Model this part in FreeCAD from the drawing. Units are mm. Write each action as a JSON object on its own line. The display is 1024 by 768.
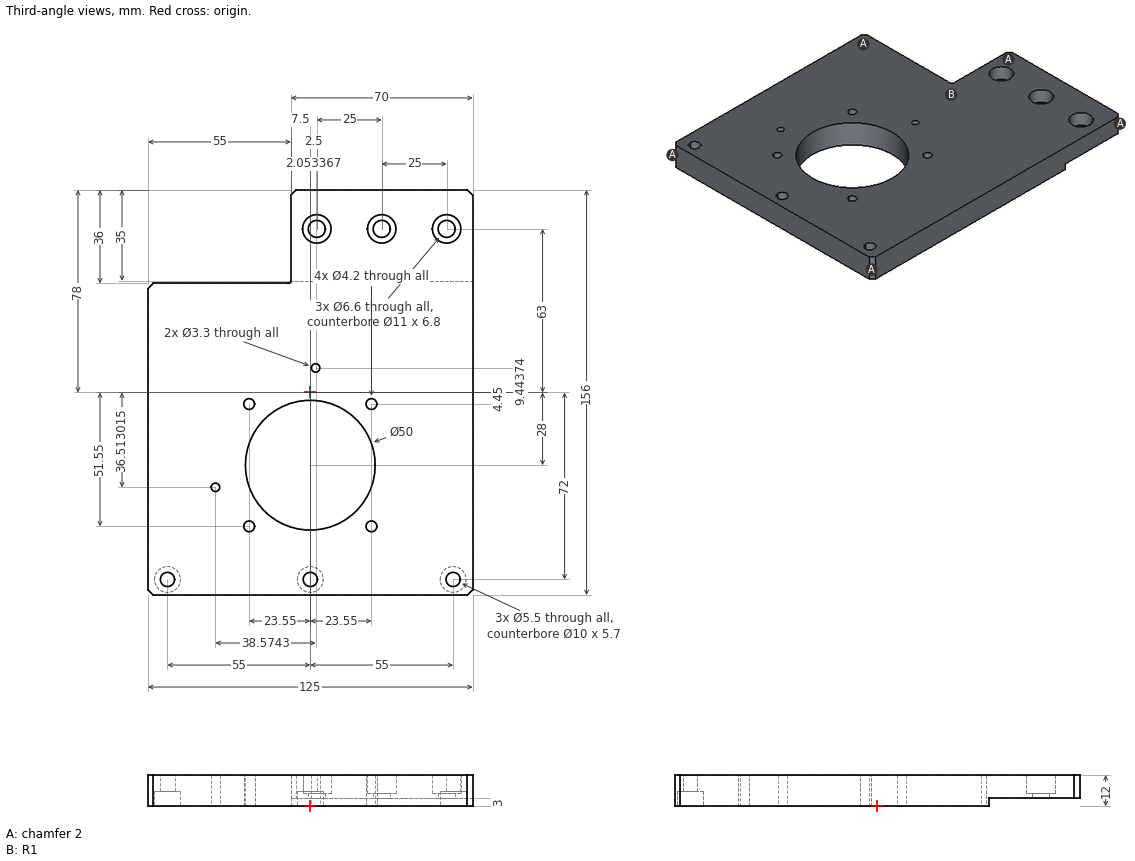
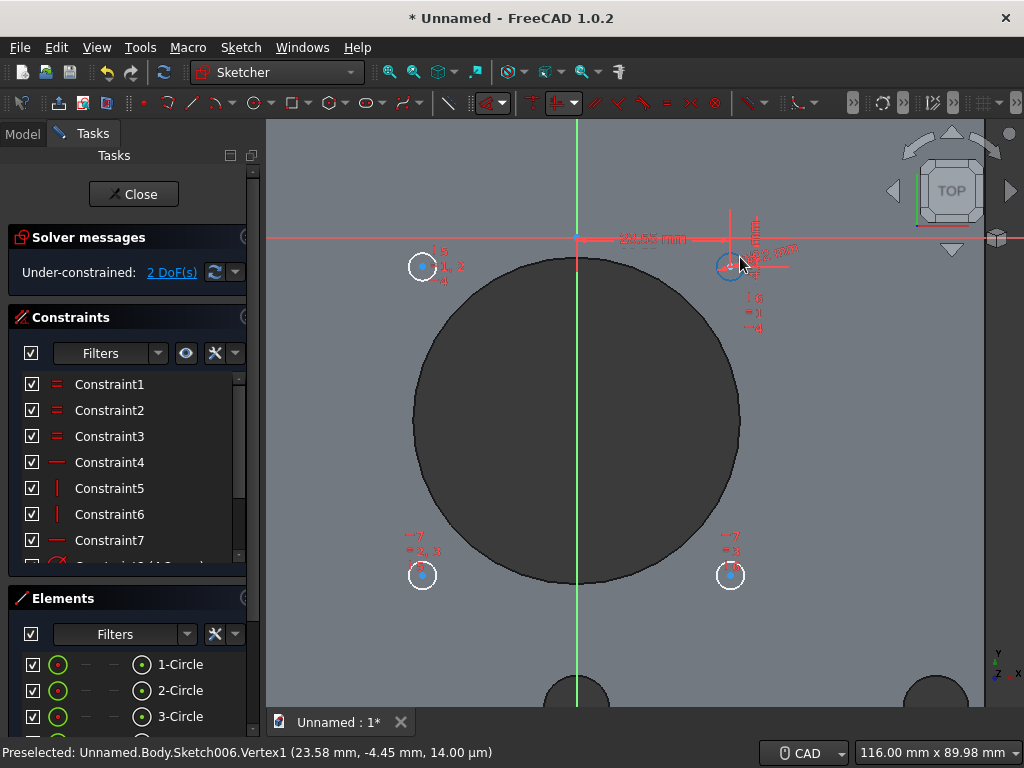
{"action": "left_click", "coordinate": [423, 267]}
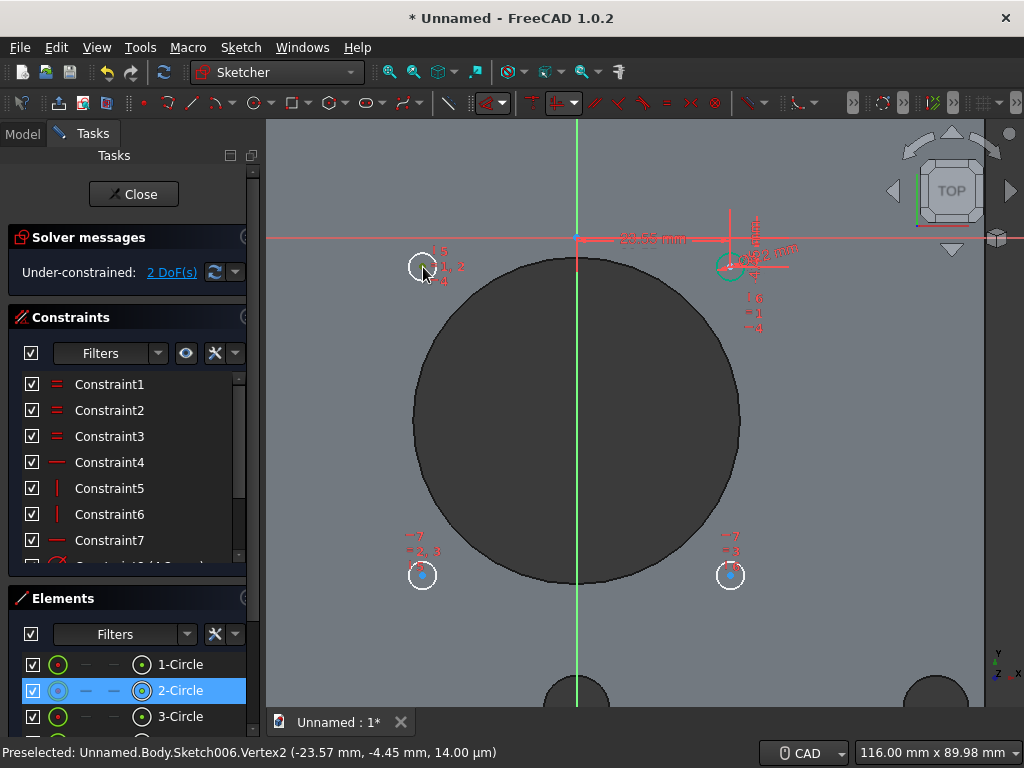
{"action": "left_click", "coordinate": [504, 104]}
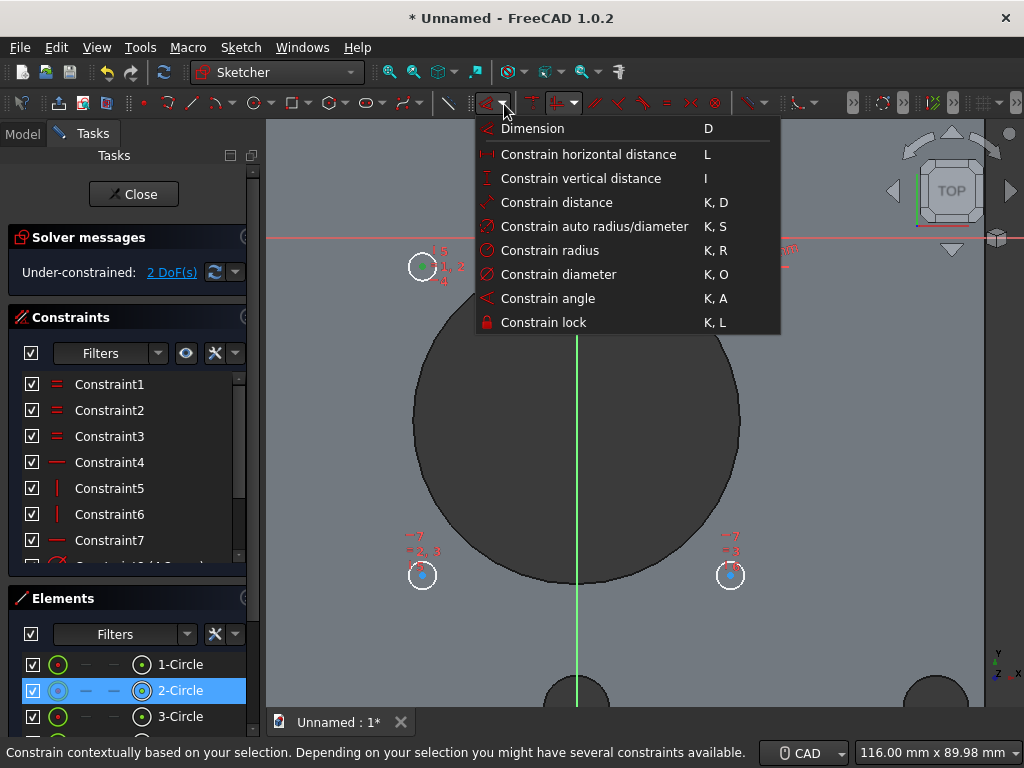
{"action": "left_click", "coordinate": [628, 154]}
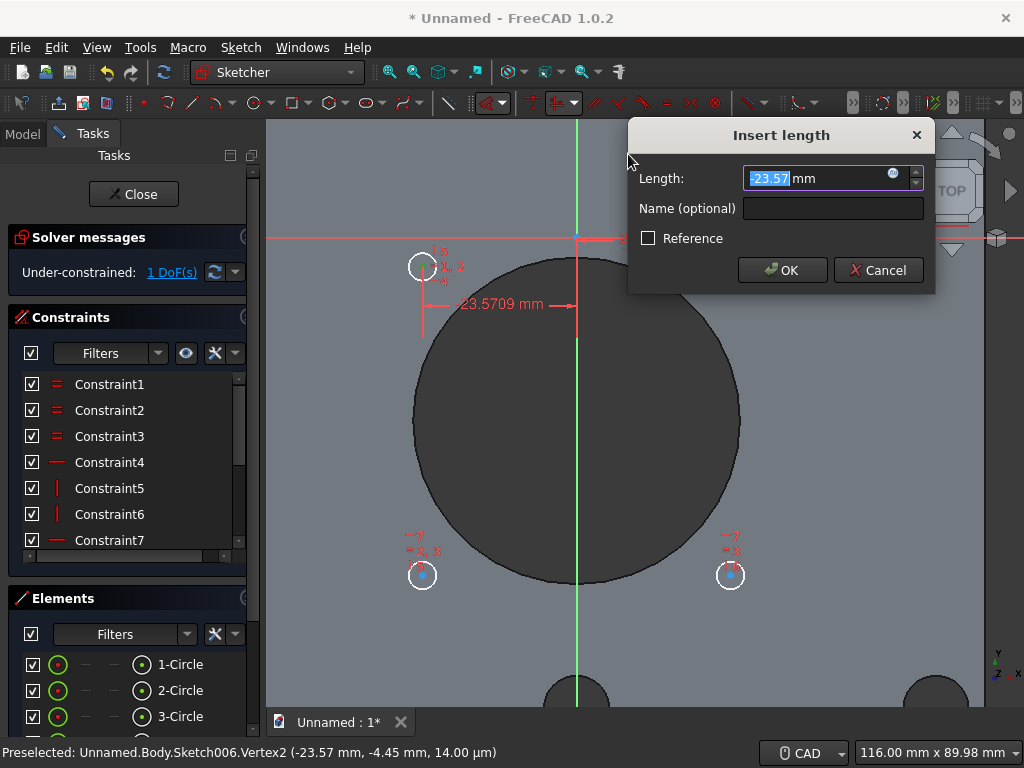
{"action": "type", "text": "-23.55"}
{"action": "key", "text": "Return"}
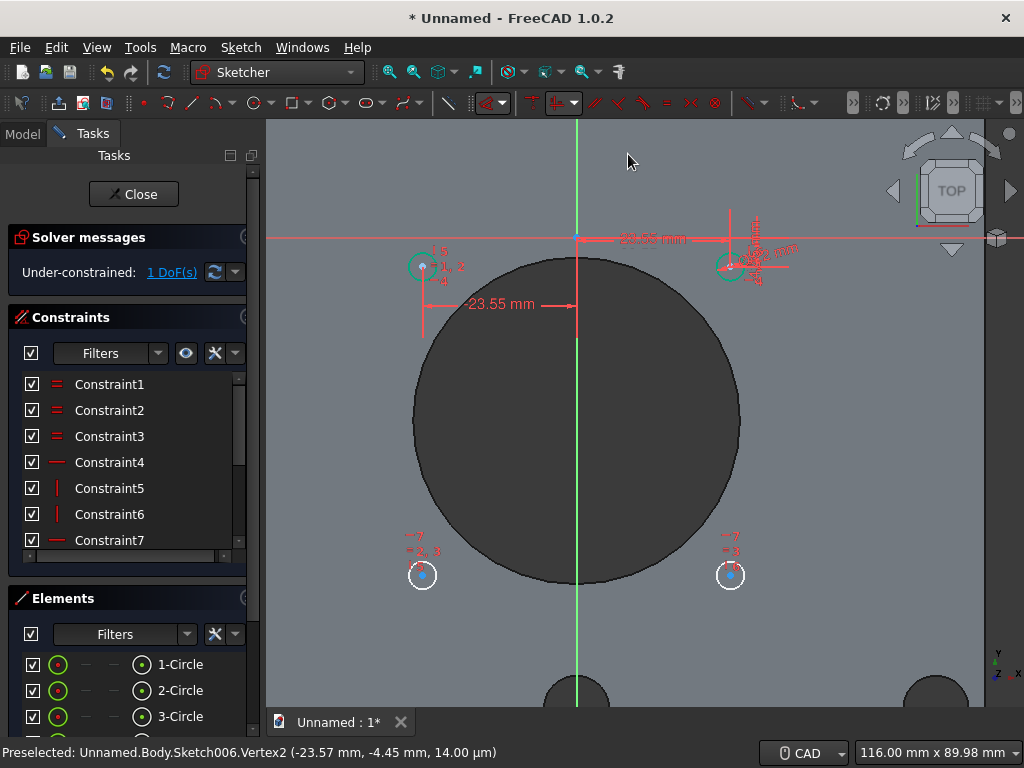
{"action": "left_click", "coordinate": [423, 575]}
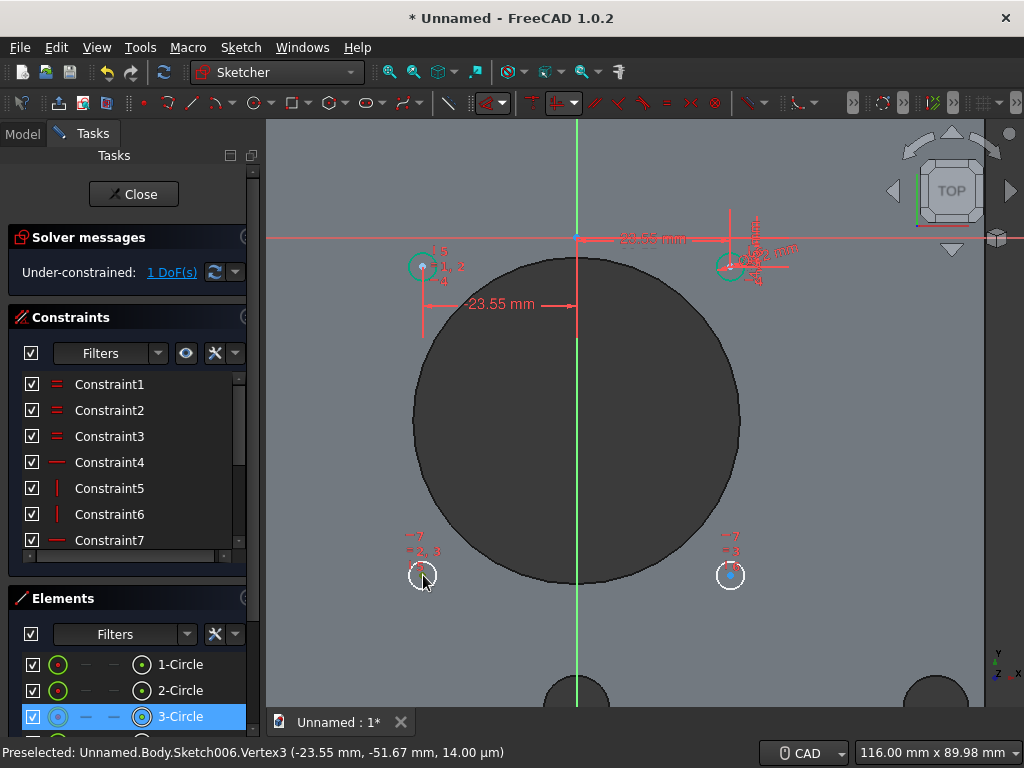
{"action": "left_click", "coordinate": [504, 104]}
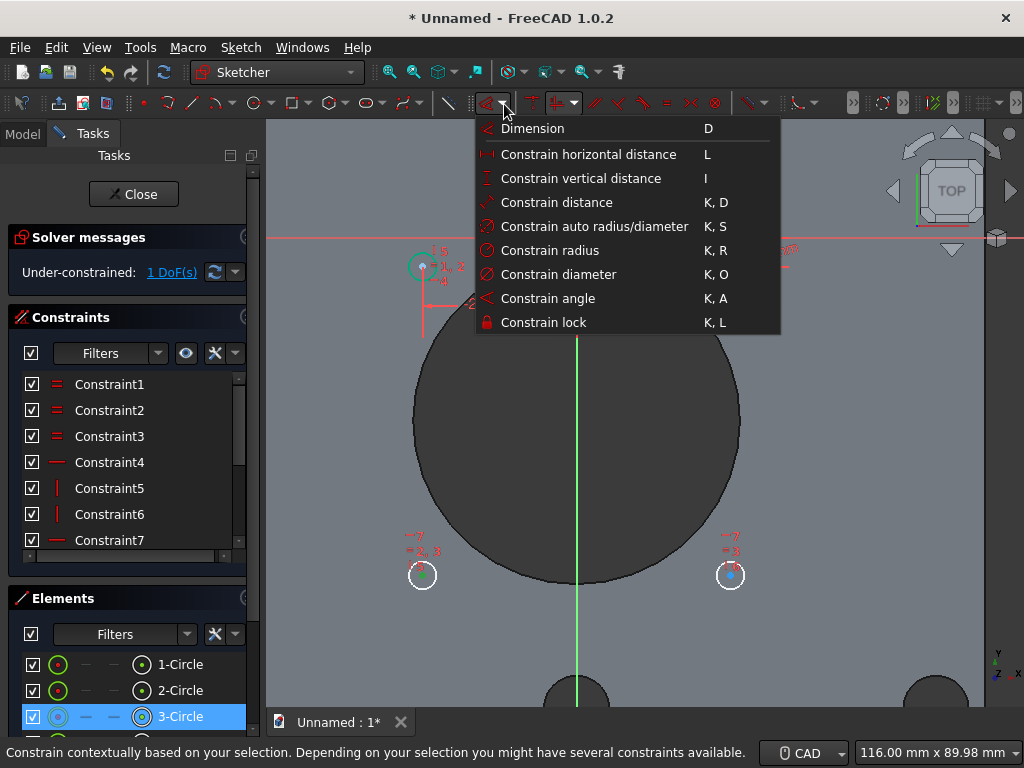
{"action": "left_click", "coordinate": [628, 178]}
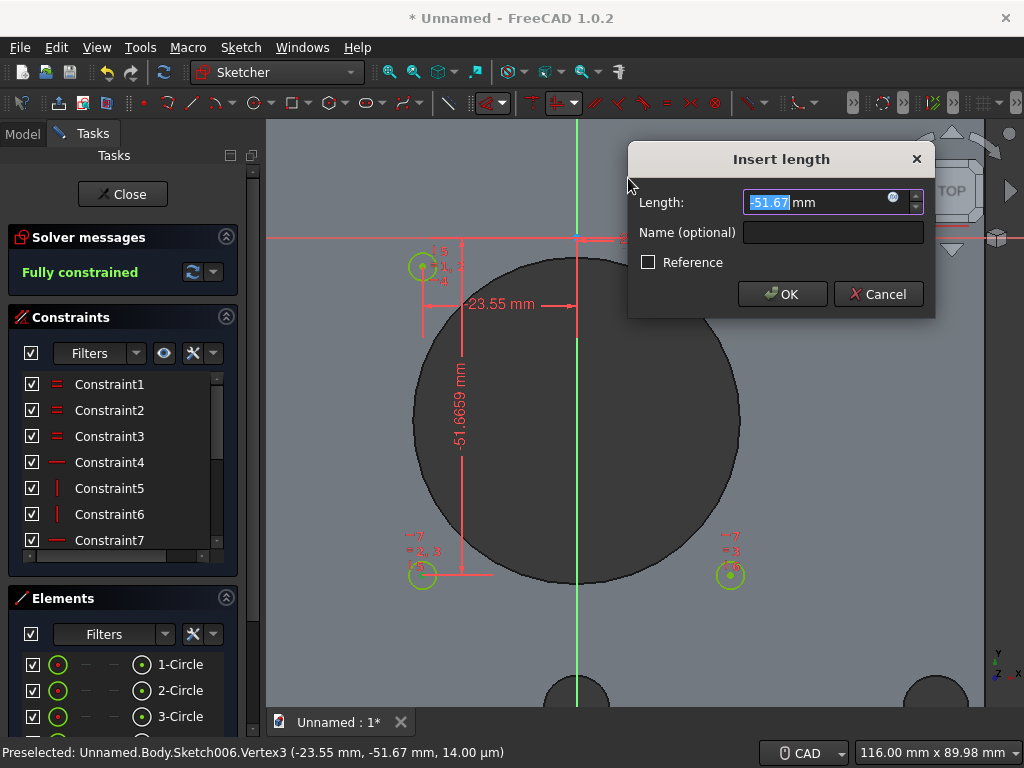
{"action": "type", "text": "-51.55"}
{"action": "key", "text": "Return"}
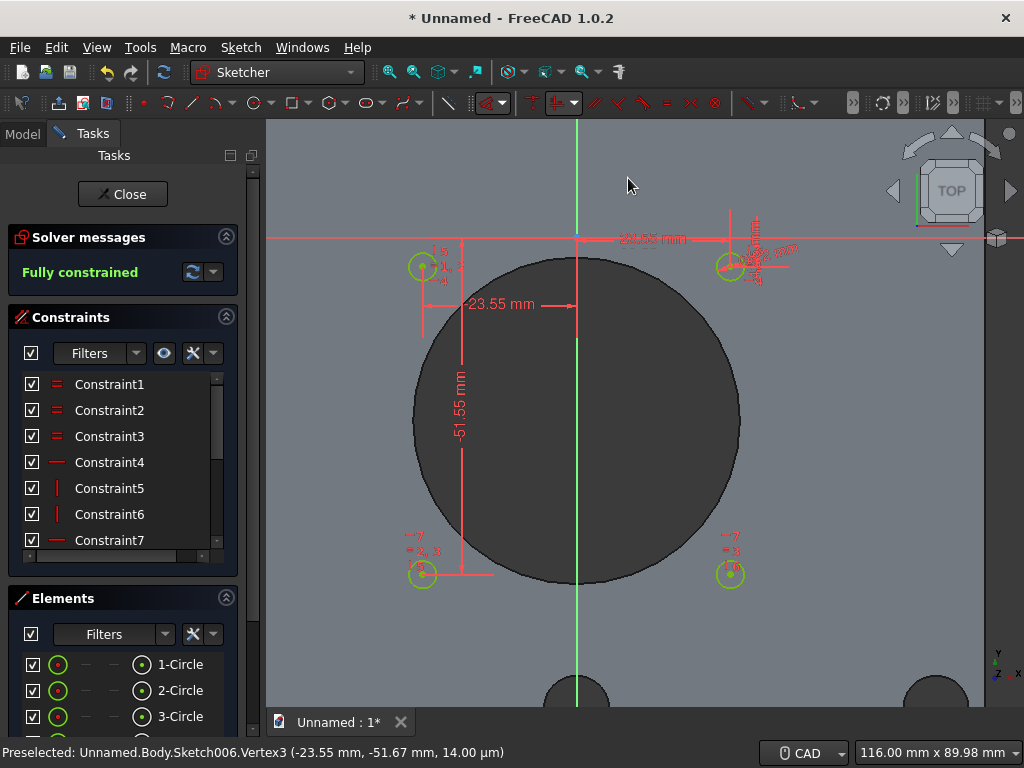
{"action": "left_click", "coordinate": [123, 194]}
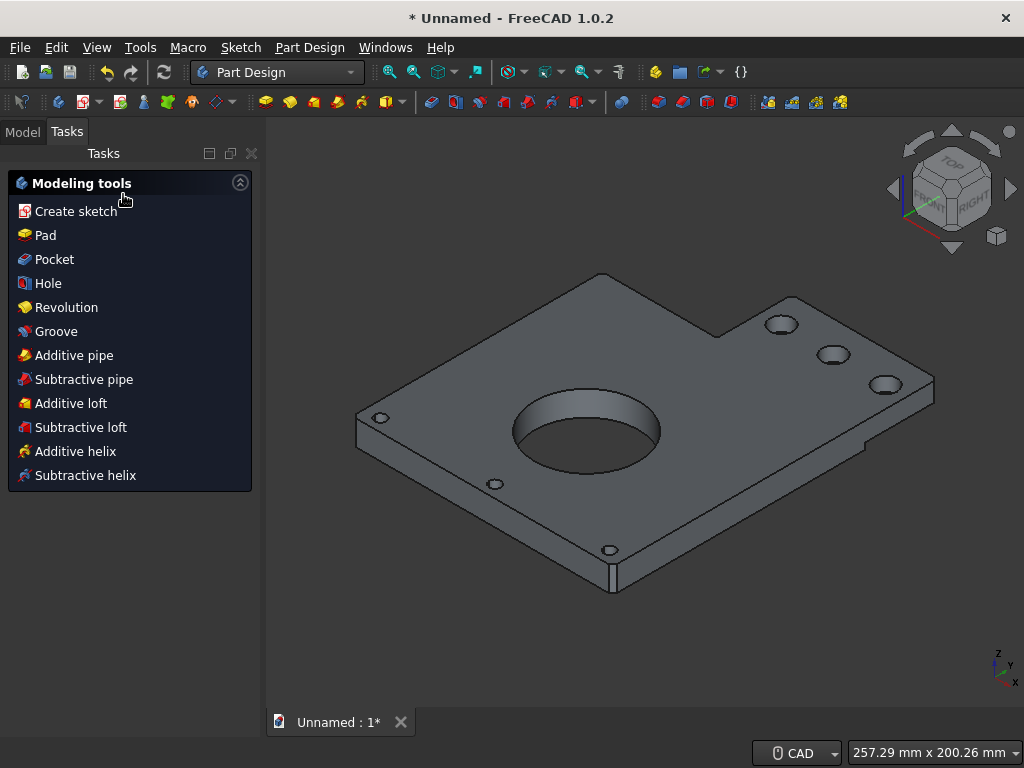
{"action": "left_click", "coordinate": [456, 102]}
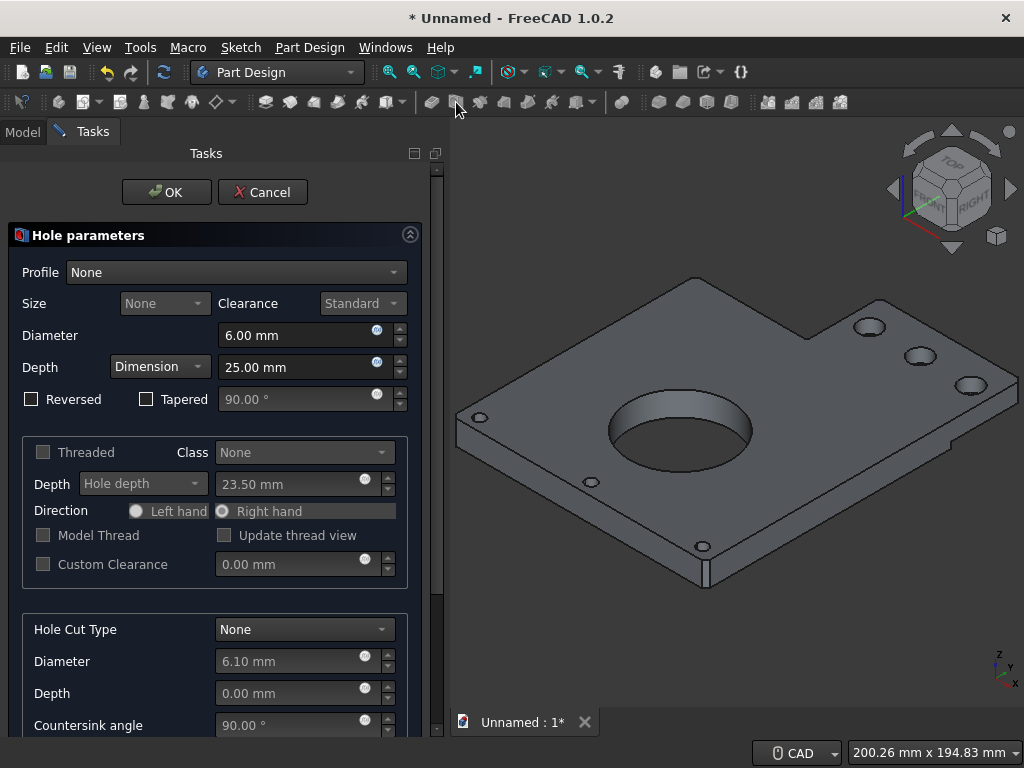
{"action": "triple_click", "coordinate": [305, 335]}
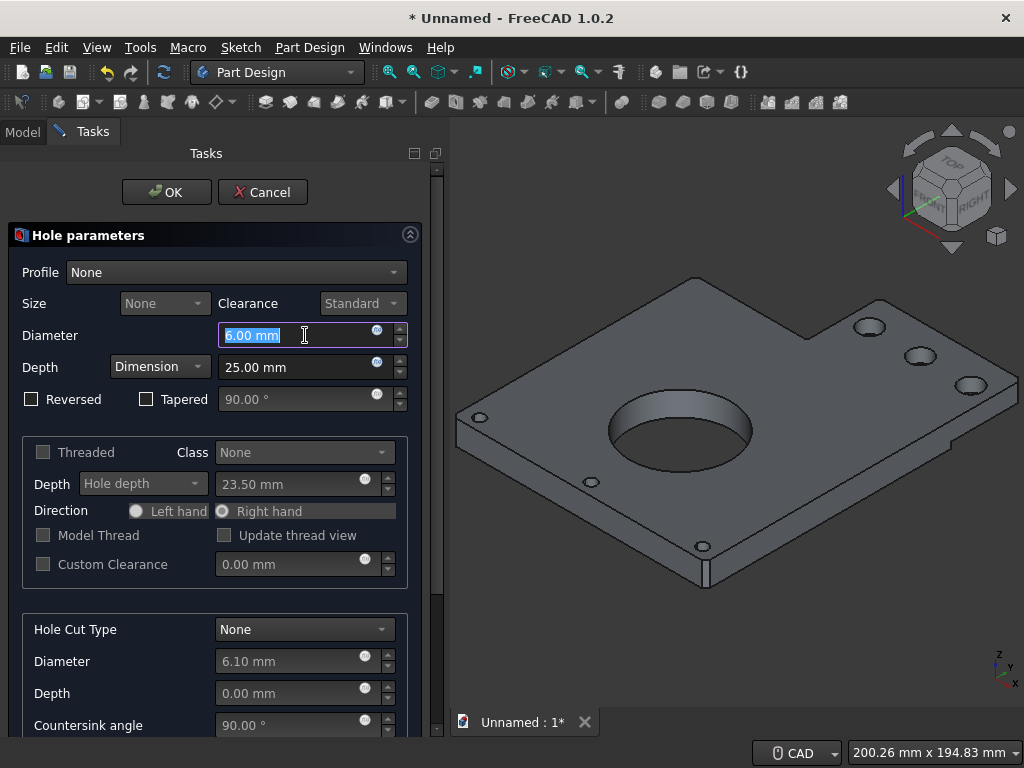
{"action": "type", "text": "4.2"}
{"action": "key", "text": "Tab"}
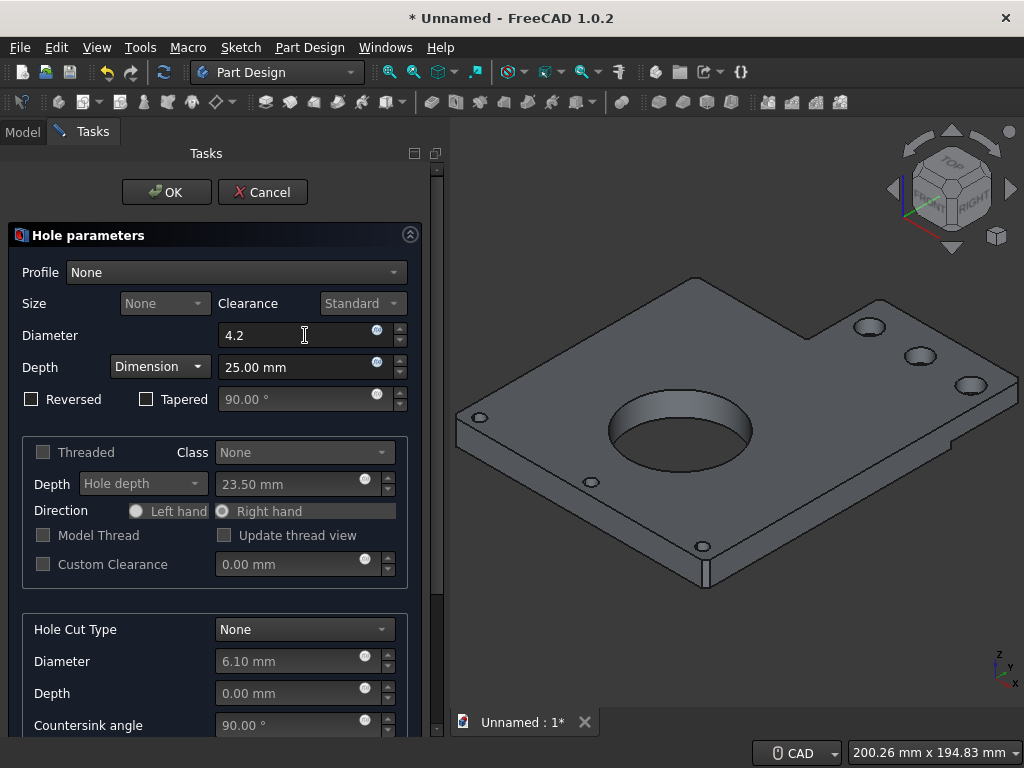
{"action": "left_click", "coordinate": [161, 366]}